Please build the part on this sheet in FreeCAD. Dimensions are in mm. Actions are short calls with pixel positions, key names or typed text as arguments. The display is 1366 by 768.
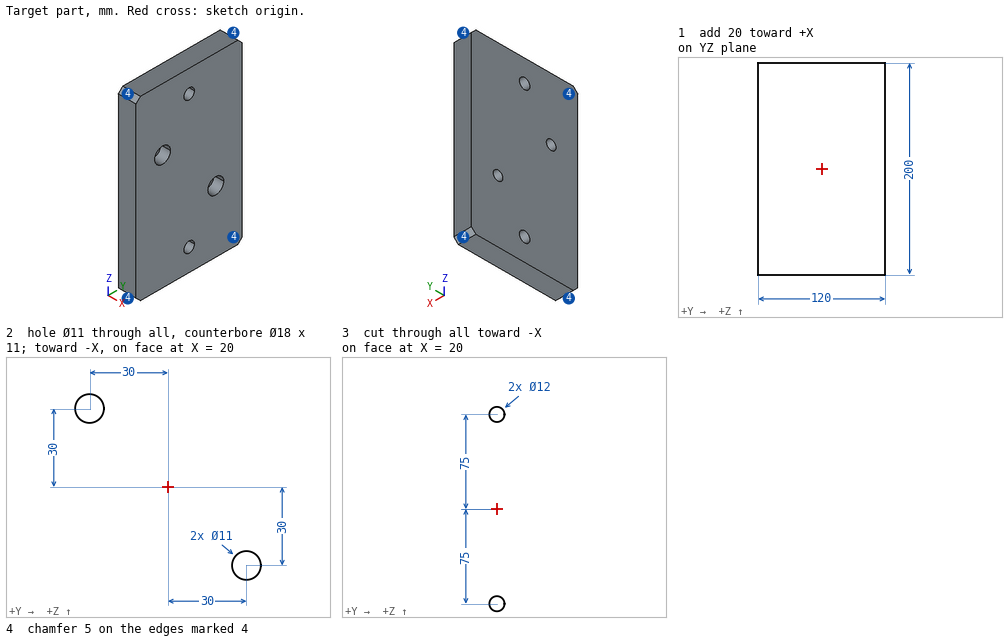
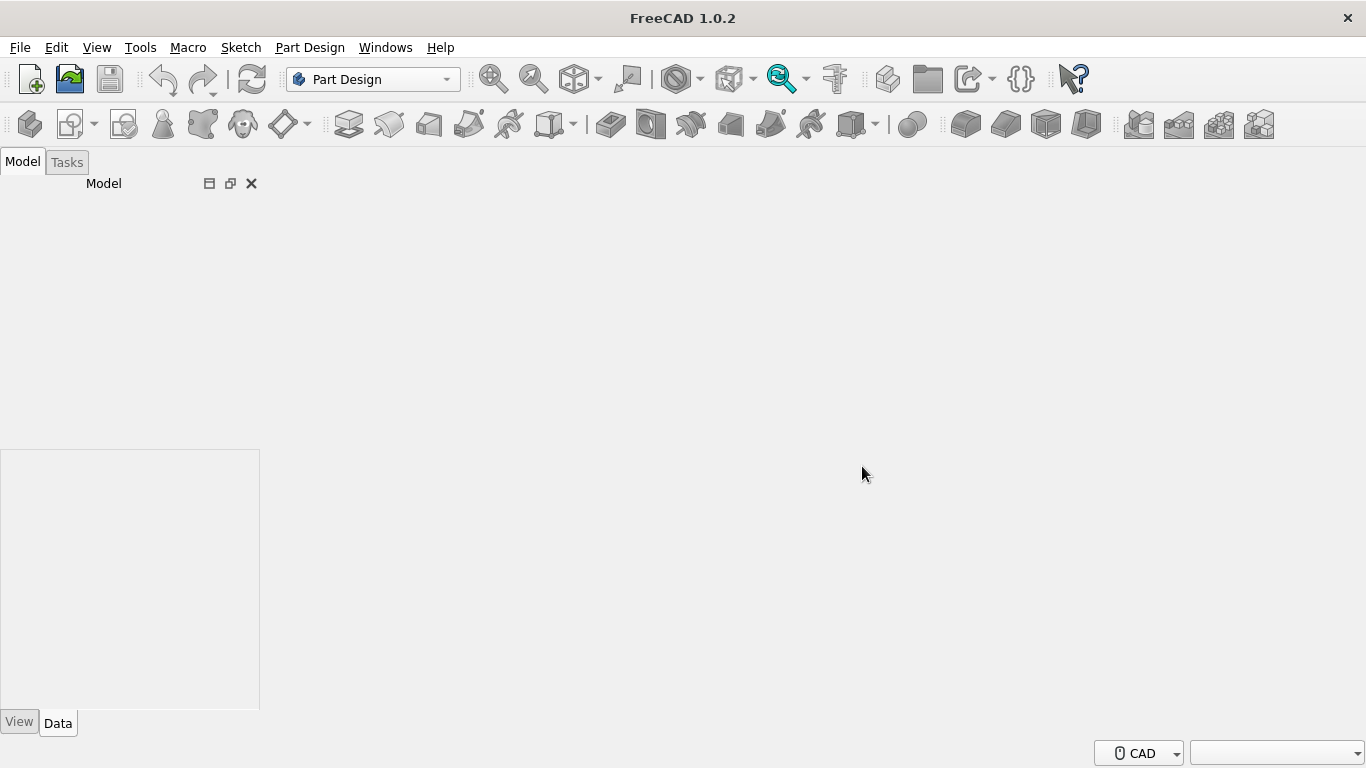
click(30, 80)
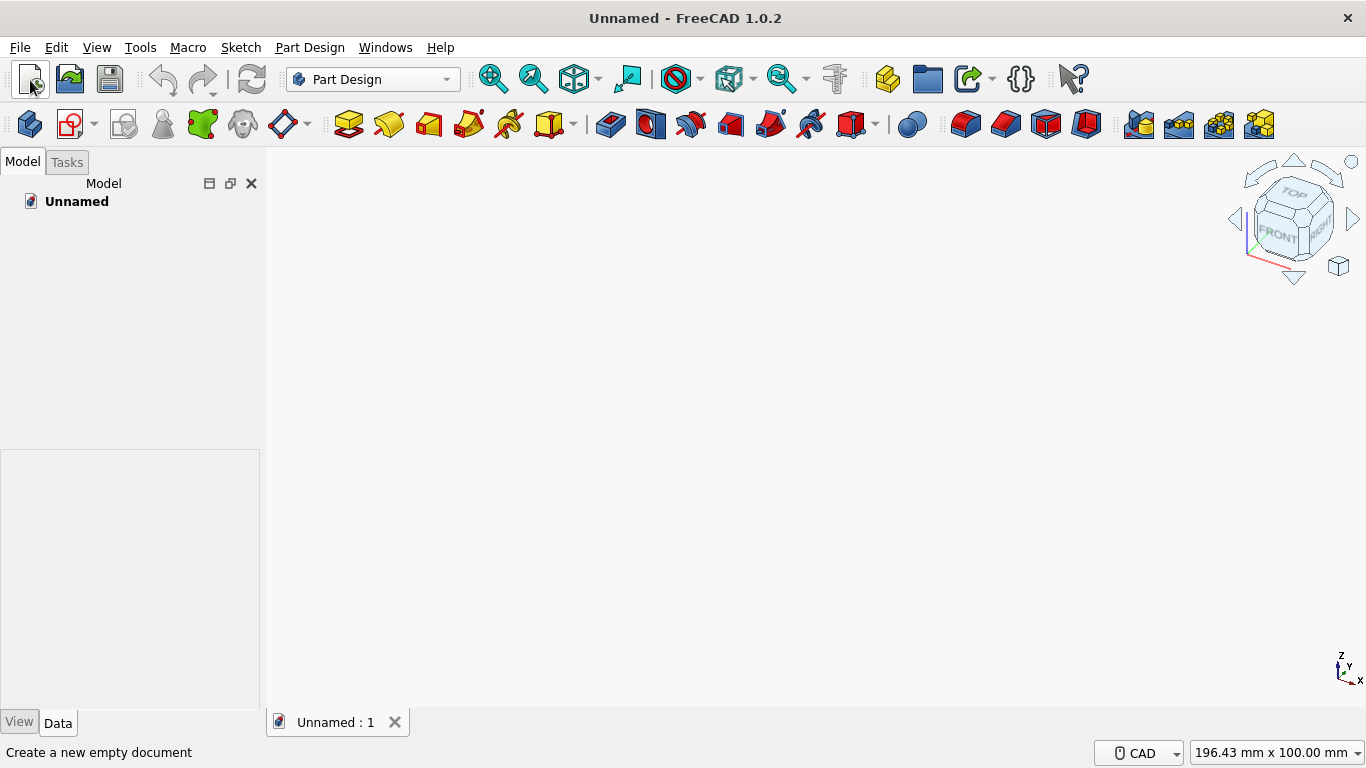
click(70, 124)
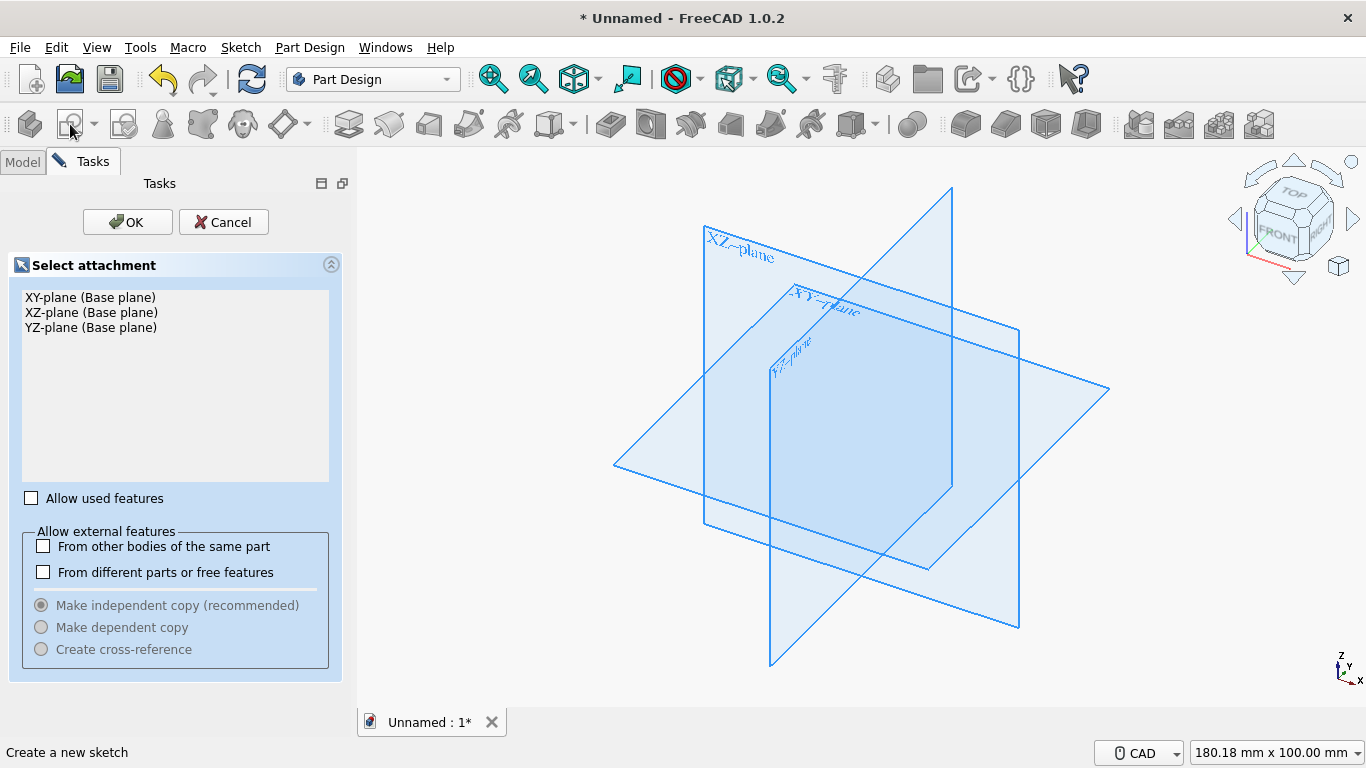
click(82, 328)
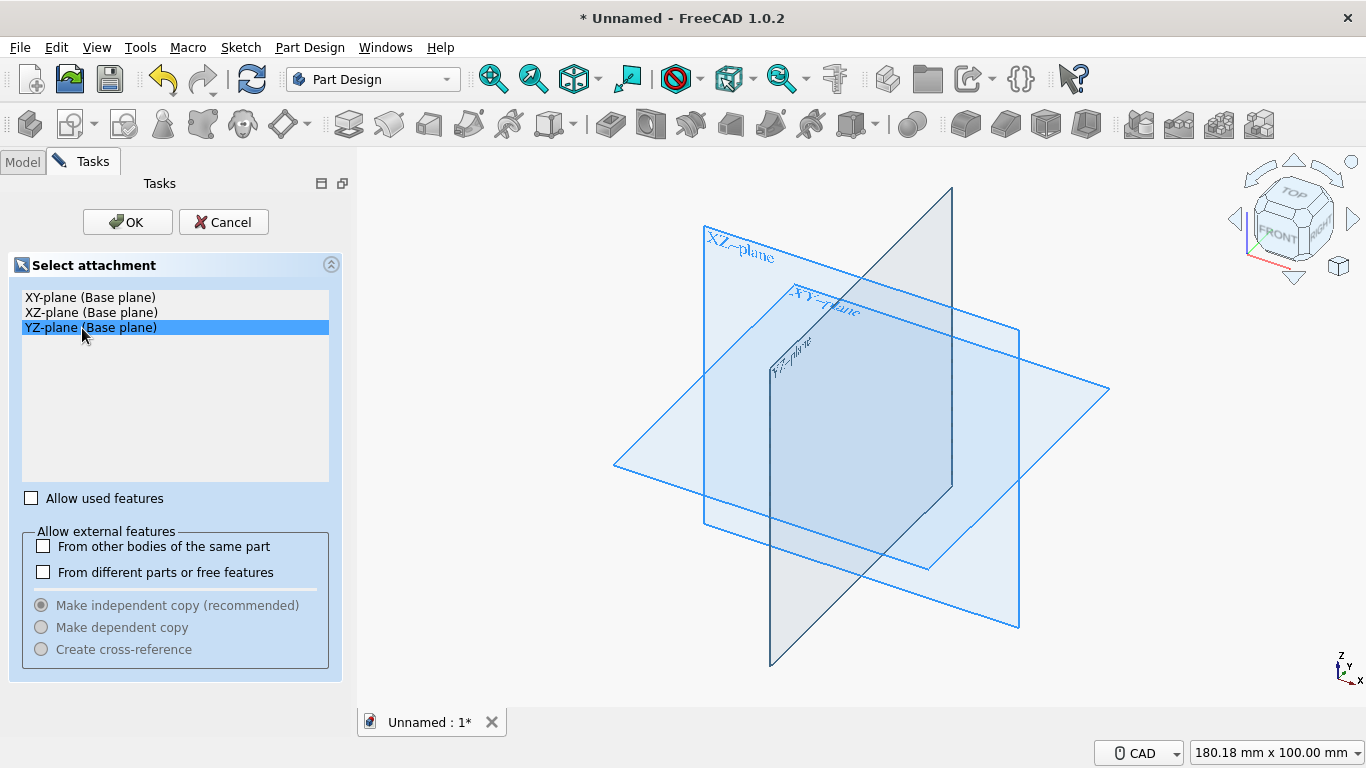
click(128, 222)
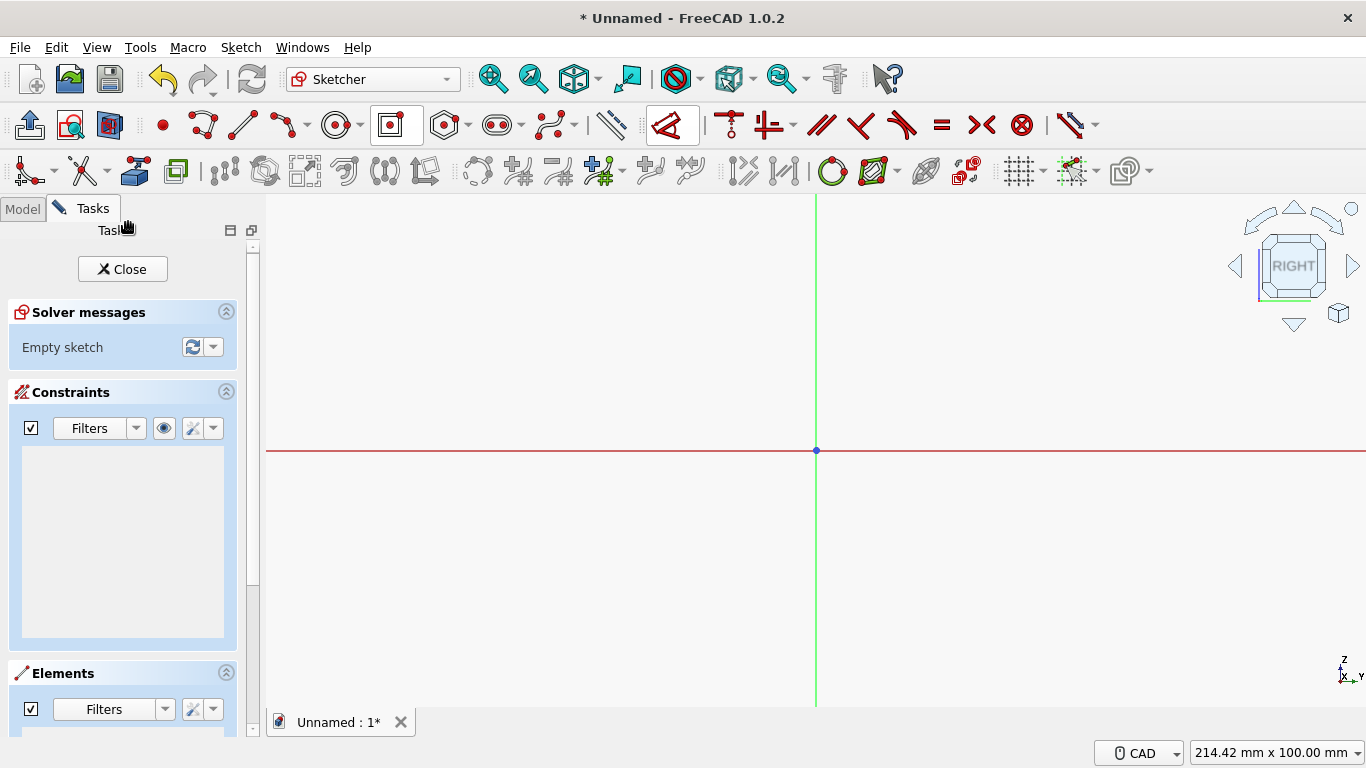
scroll(718, 450, down, 6)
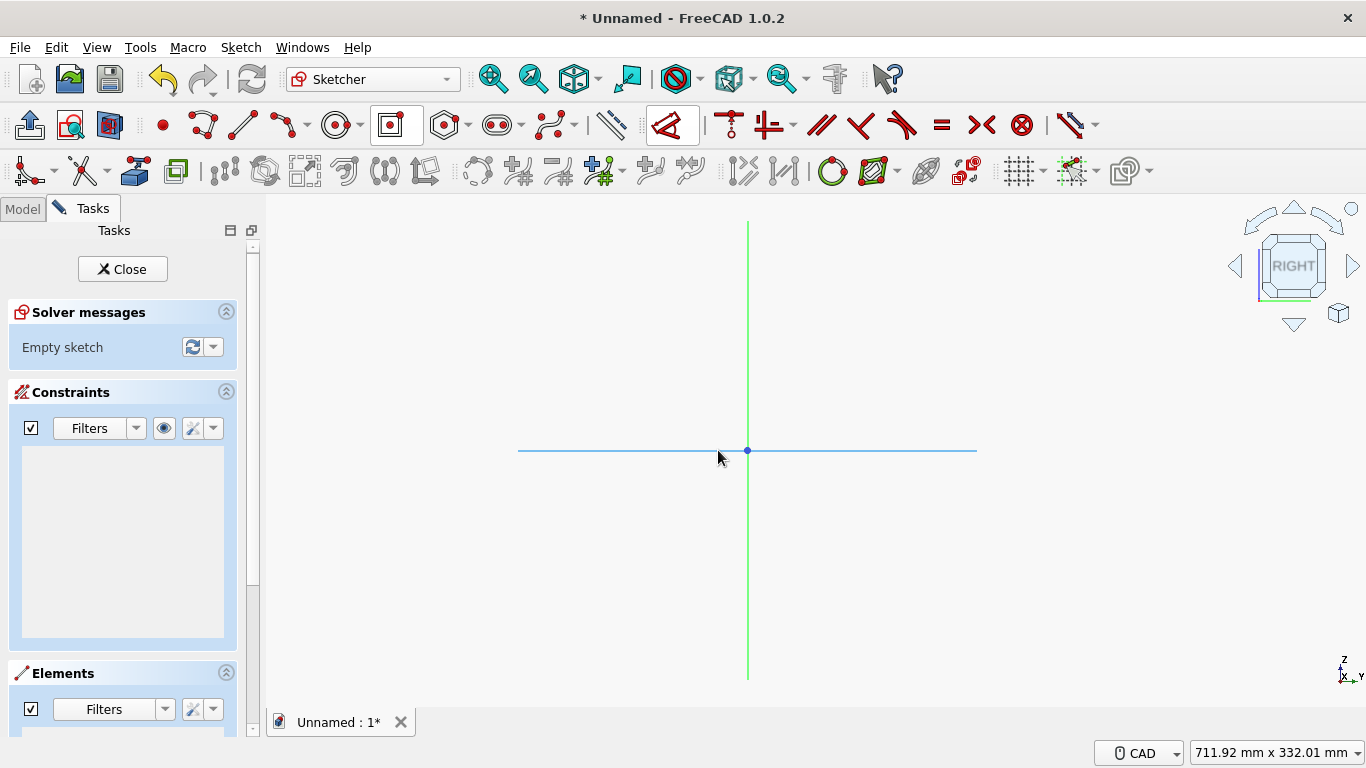
click(390, 126)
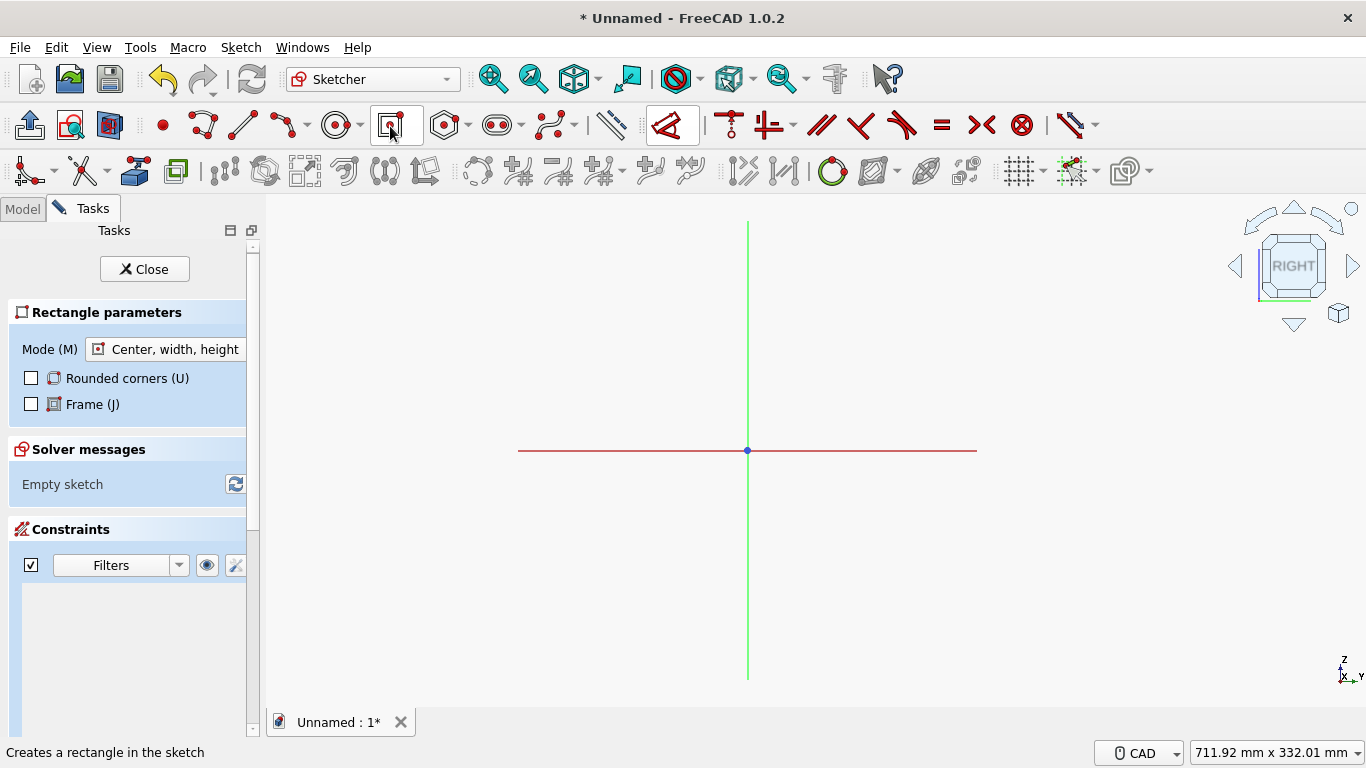
click(748, 450)
move(841, 296)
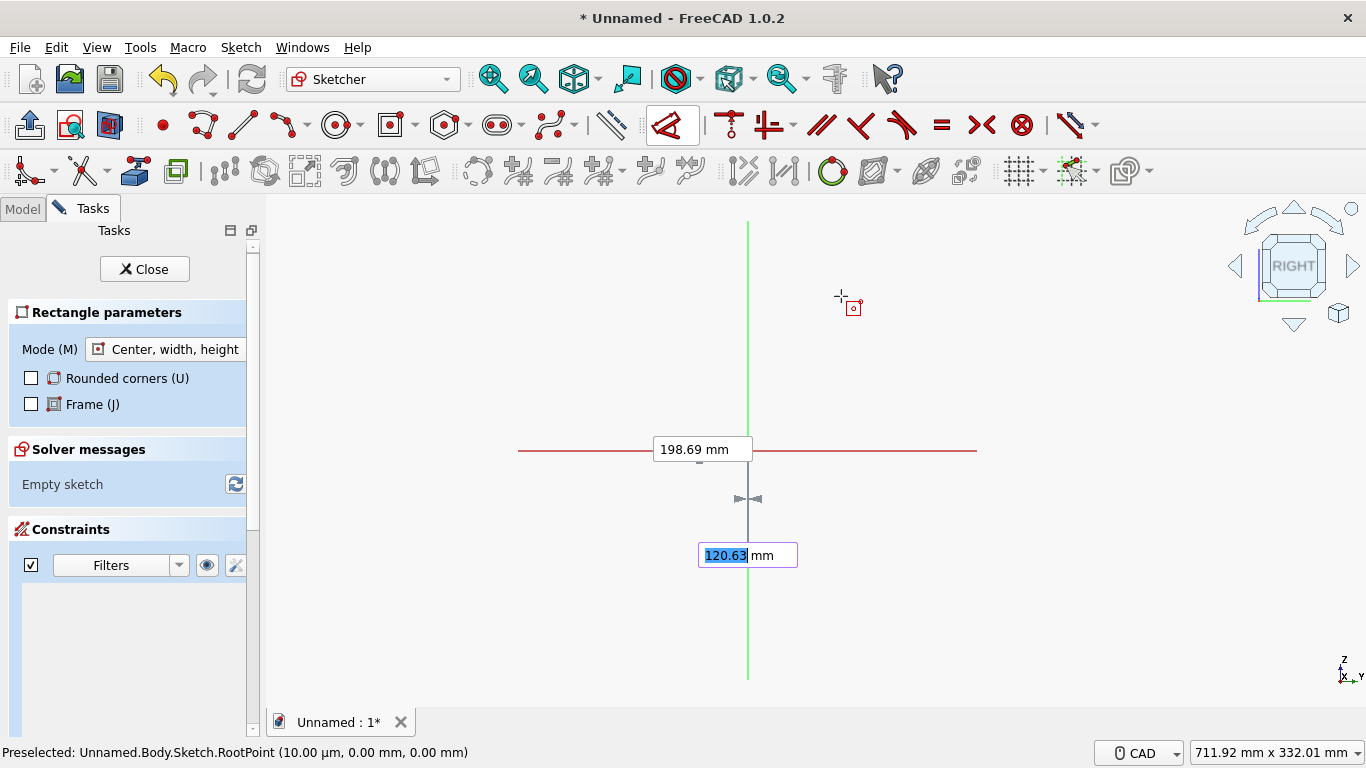
text(120)
key(Tab)
text(200)
key(Return)
key(Escape)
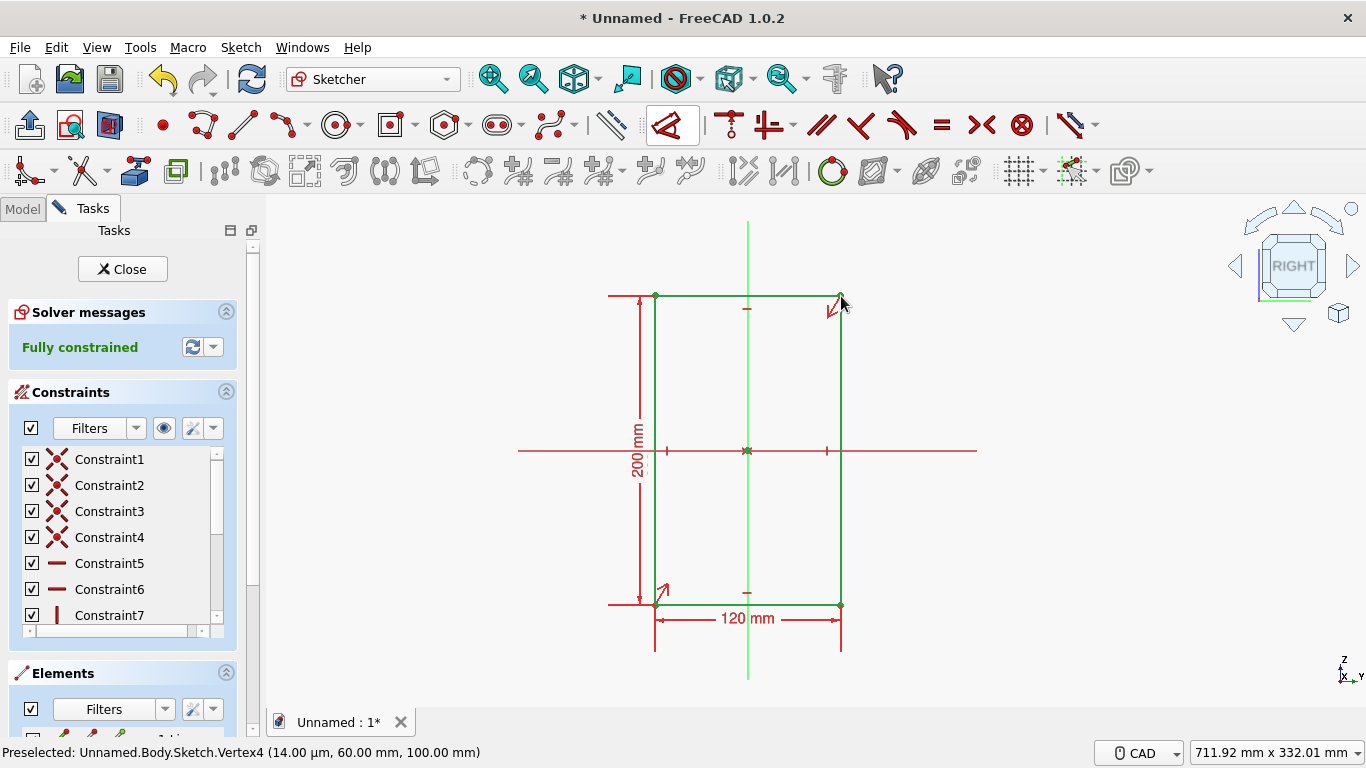
click(123, 269)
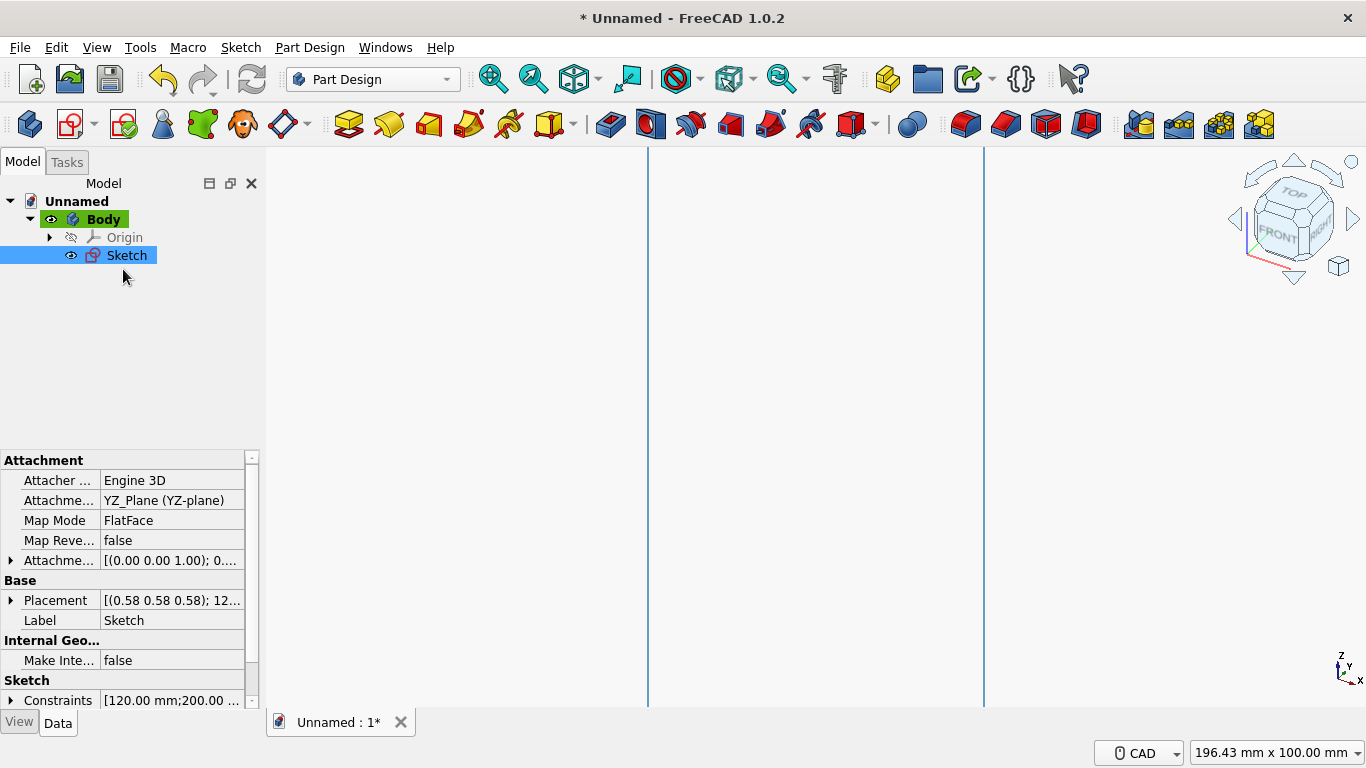
click(350, 124)